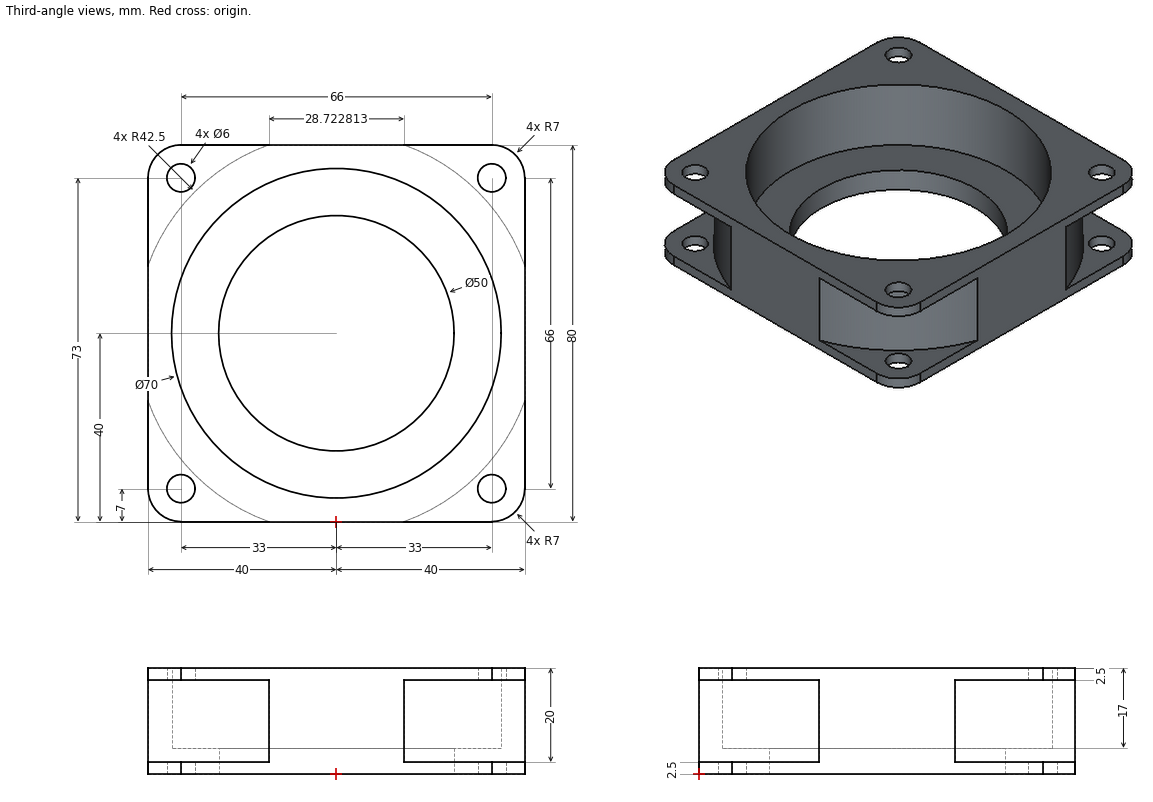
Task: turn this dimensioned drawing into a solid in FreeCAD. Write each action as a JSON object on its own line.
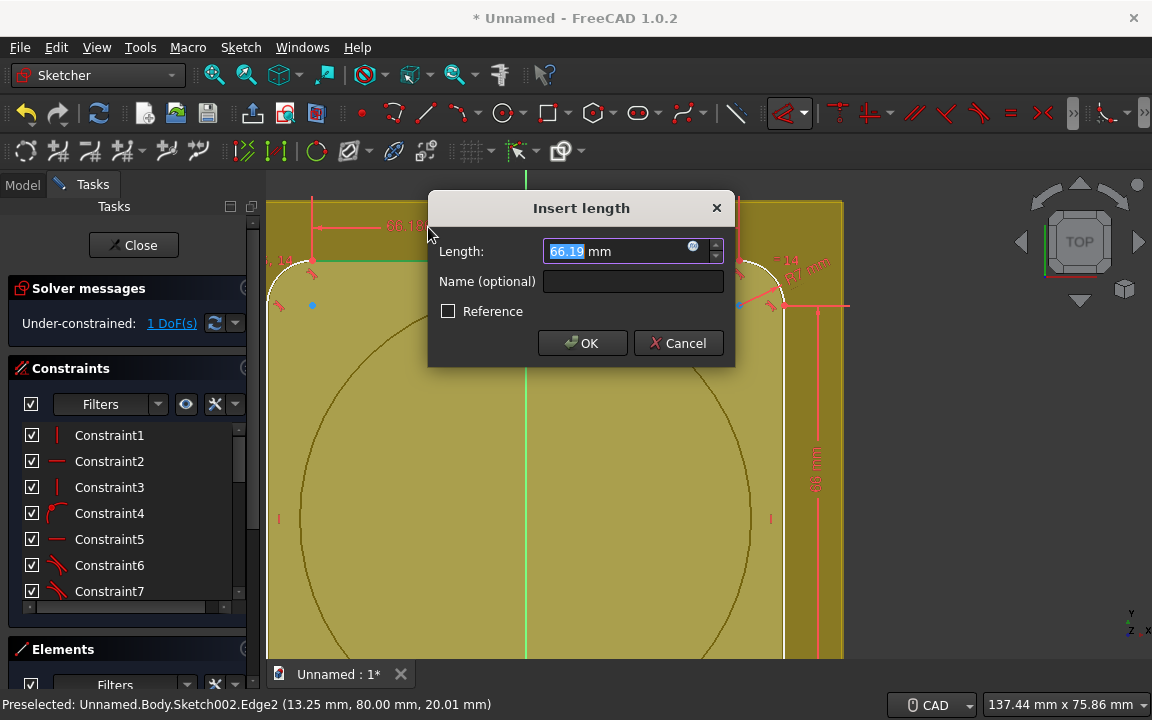
{"action": "type", "text": "66"}
{"action": "key", "text": "Return"}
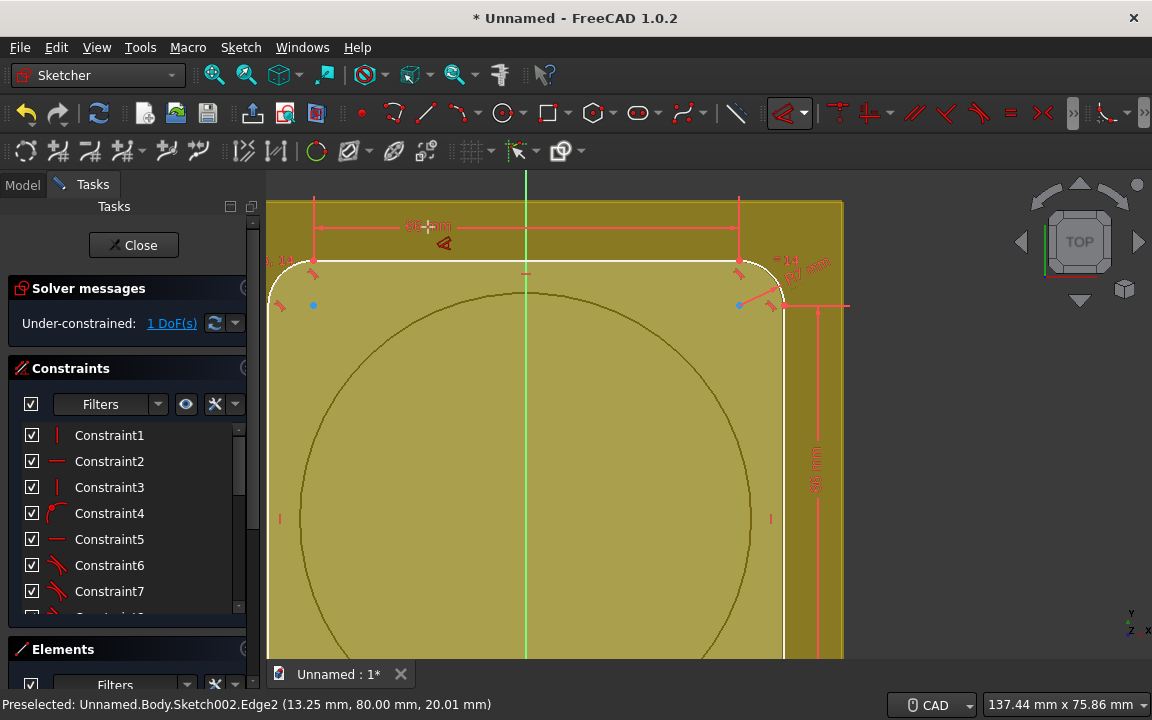
{"action": "scroll", "coordinate": [780, 288], "scroll_direction": "down", "scroll_amount": 3}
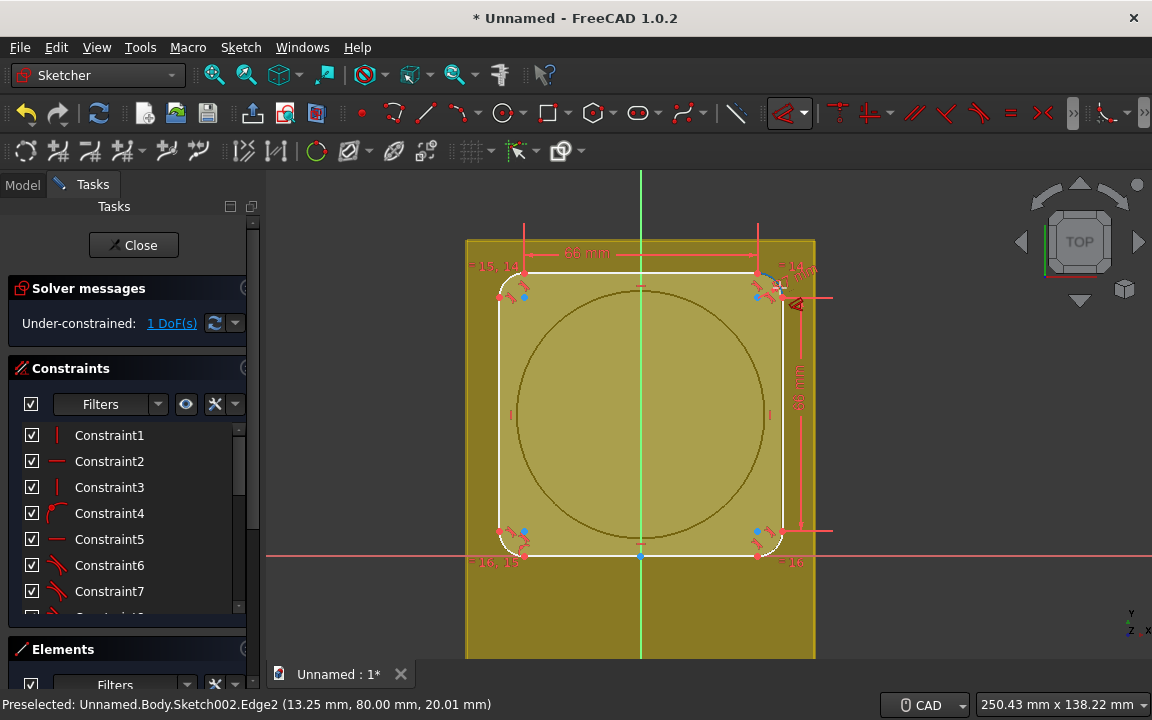
{"action": "left_click", "coordinate": [783, 531]}
{"action": "left_click", "coordinate": [712, 590]}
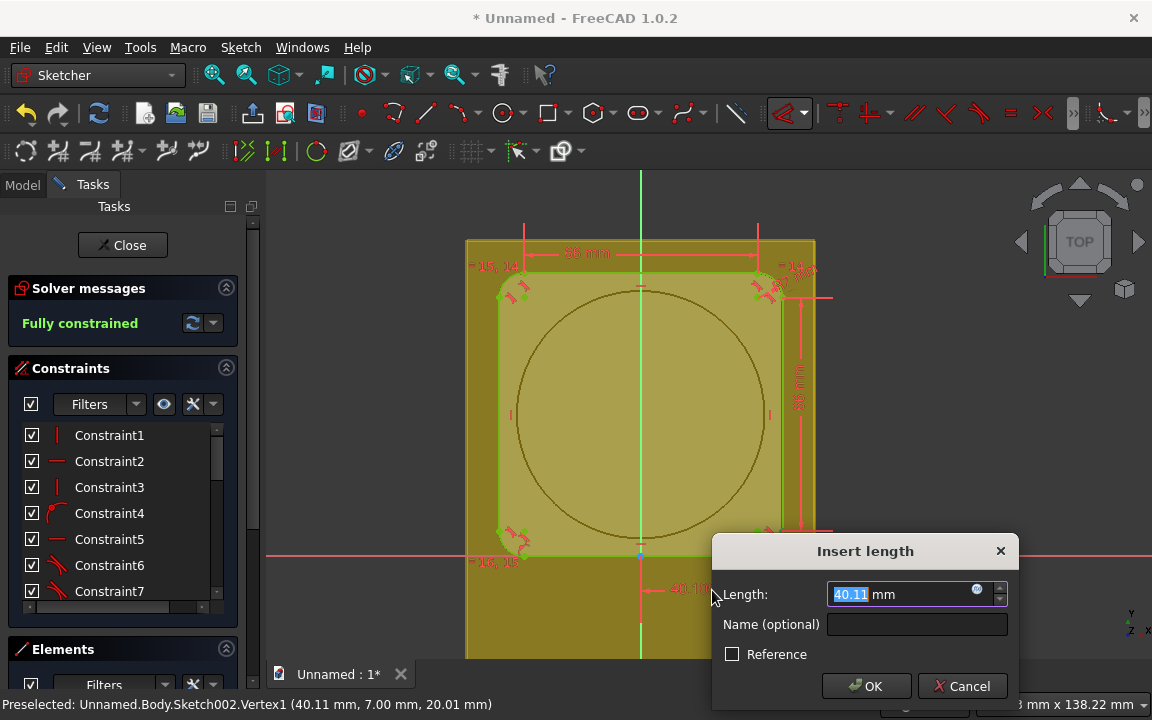
{"action": "type", "text": "40"}
{"action": "key", "text": "Return"}
{"action": "key", "text": "Escape"}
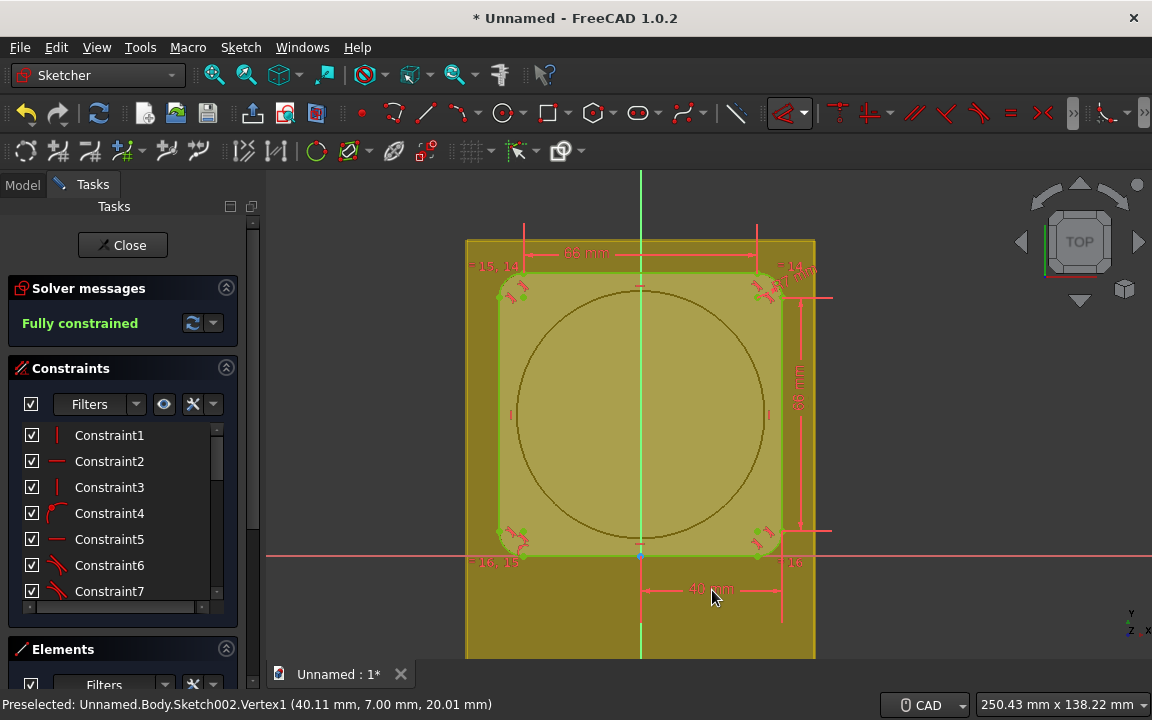
{"action": "left_click", "coordinate": [123, 245]}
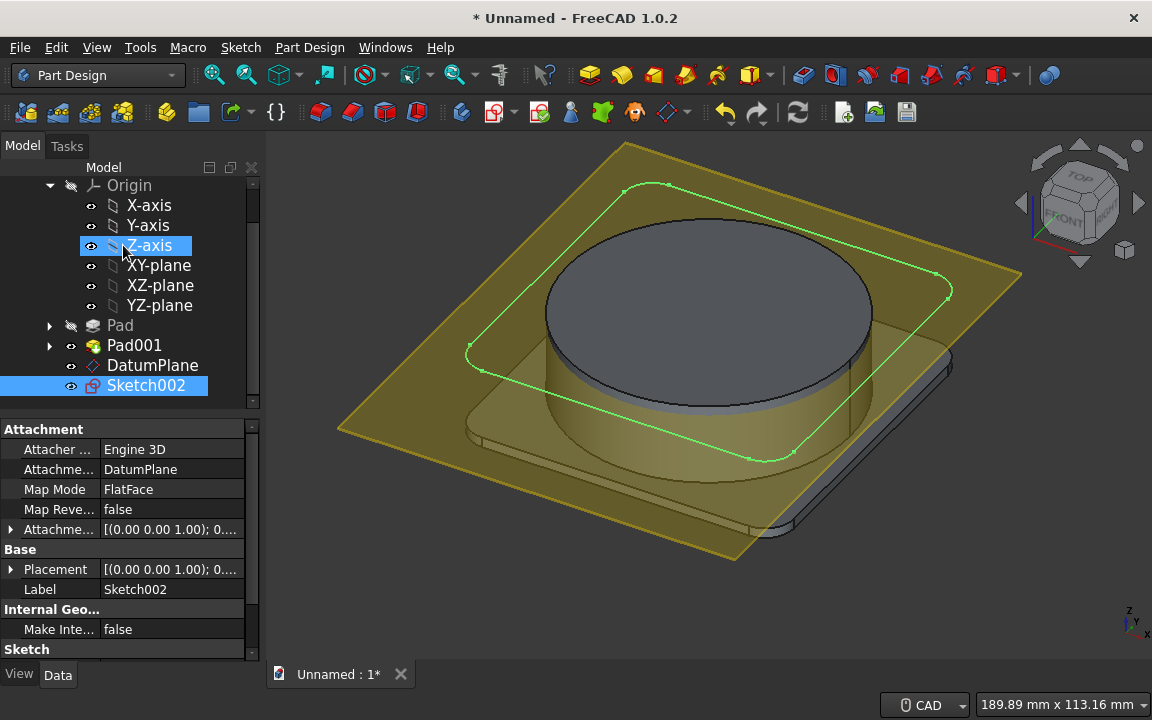
{"action": "left_click", "coordinate": [590, 76]}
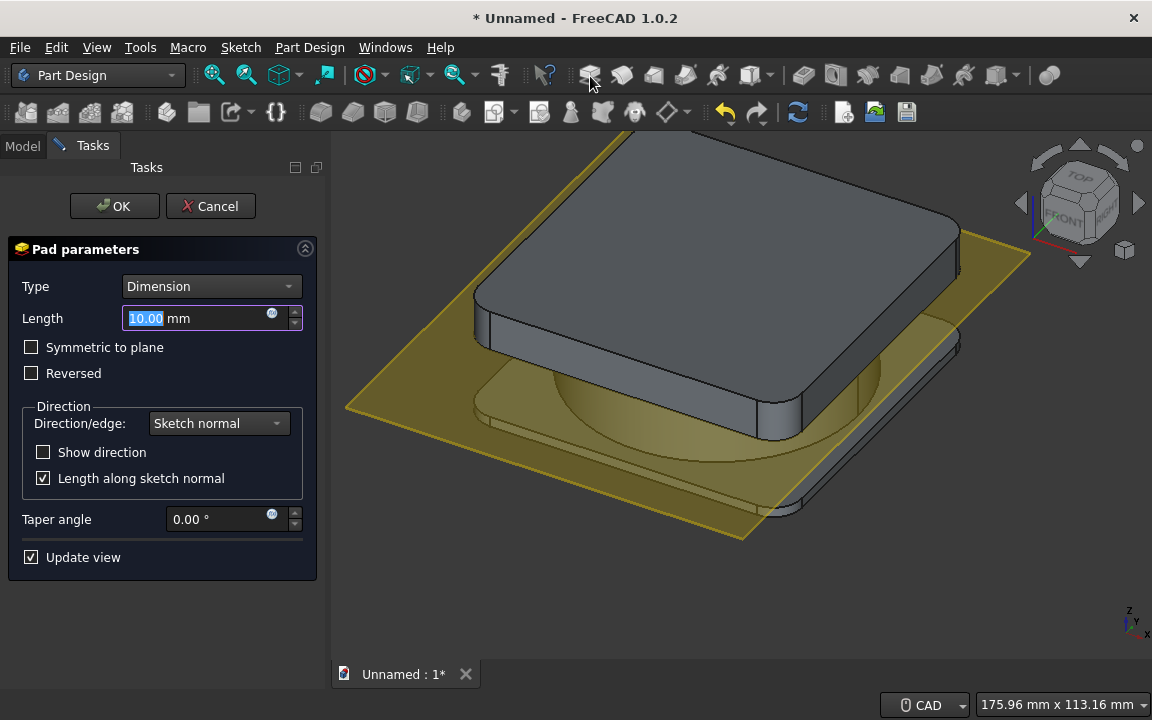
{"action": "type", "text": "2.5"}
{"action": "key", "text": "Tab"}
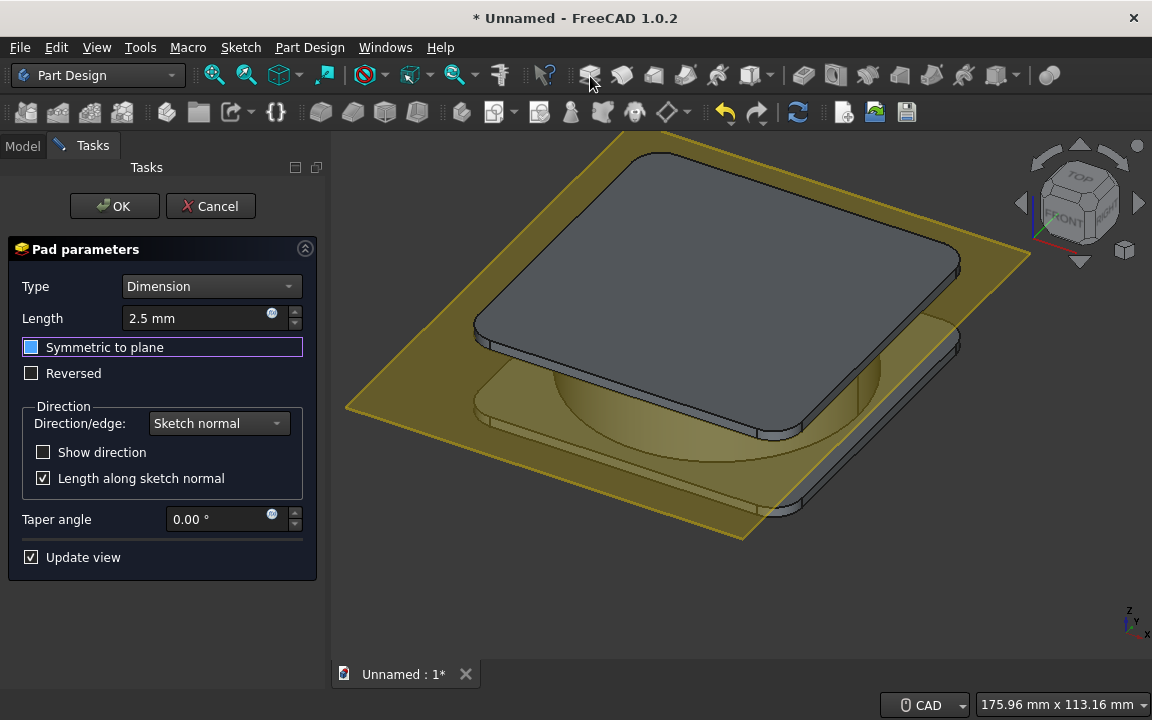
{"action": "left_click", "coordinate": [115, 206]}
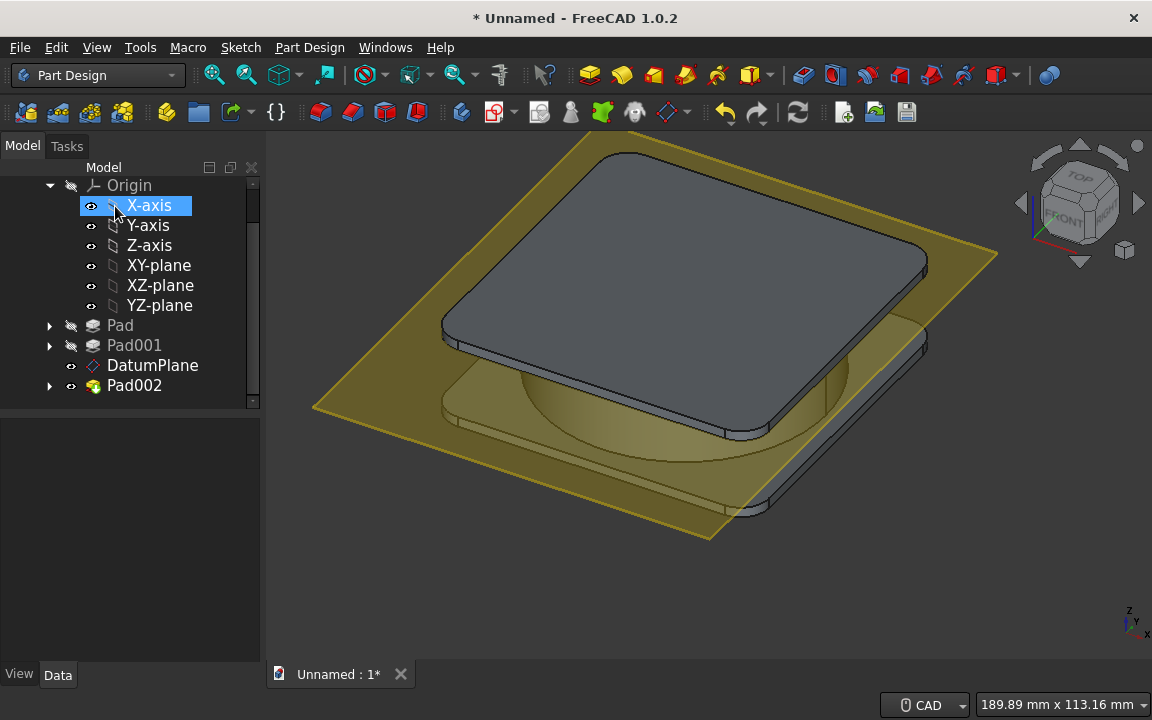
{"action": "left_click", "coordinate": [116, 366]}
{"action": "key", "text": "space"}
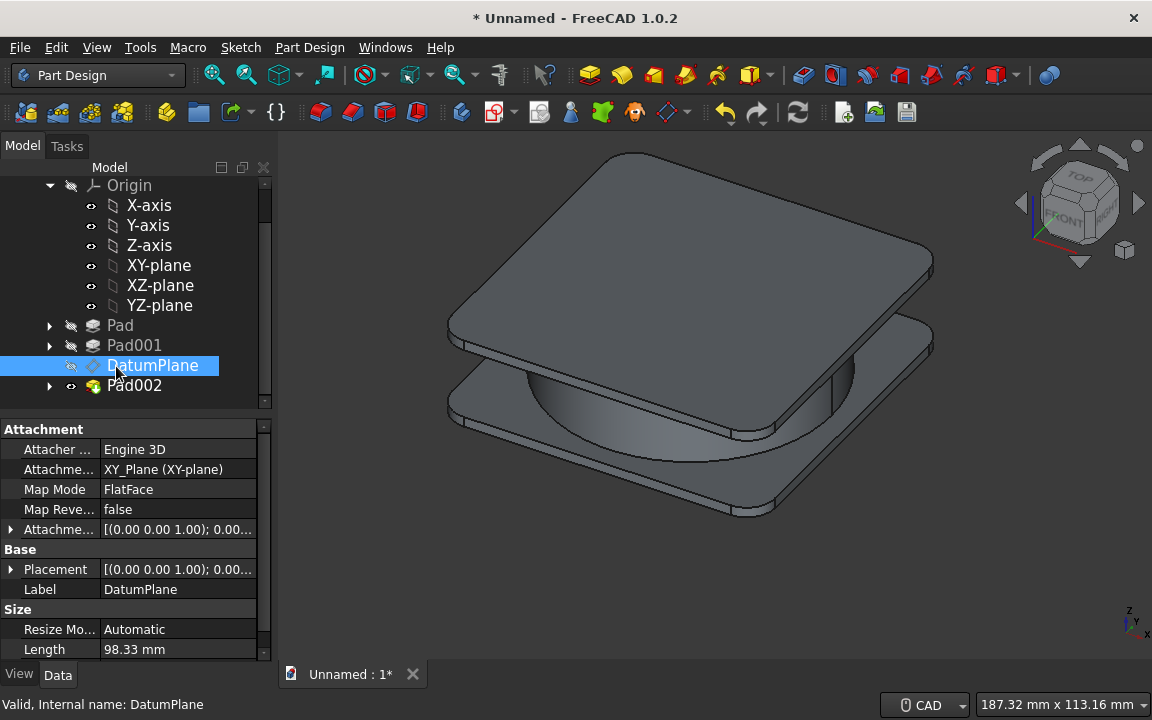
{"action": "left_click", "coordinate": [691, 291]}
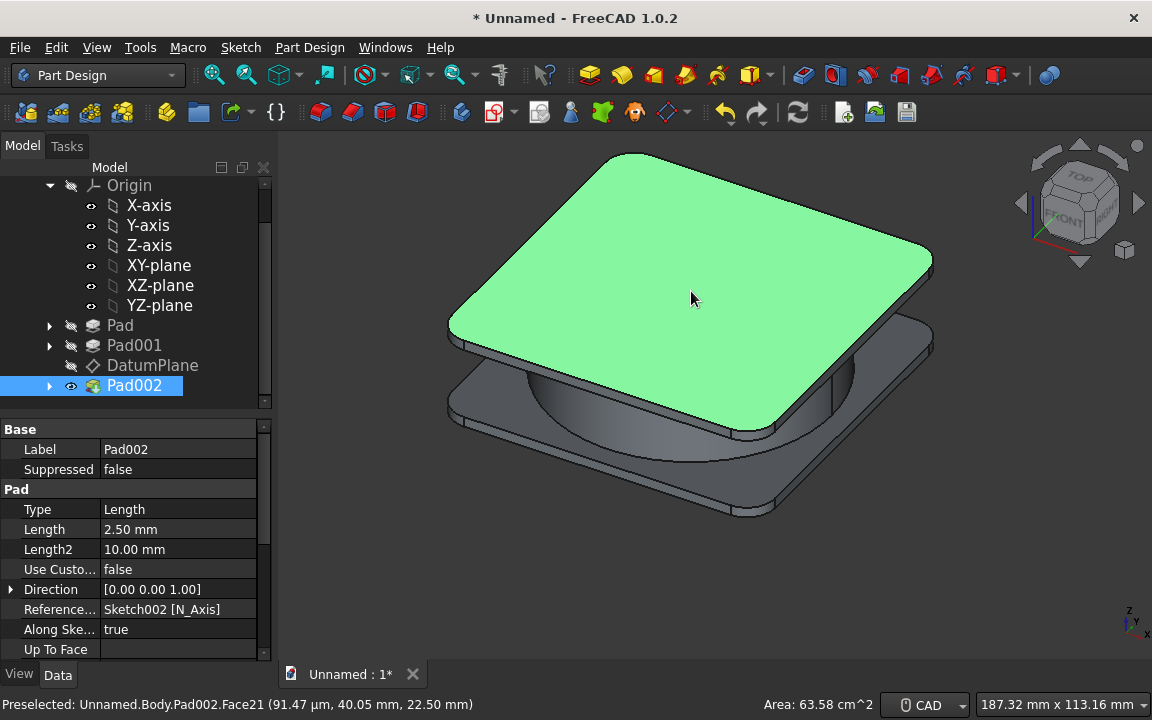
{"action": "left_click", "coordinate": [494, 112]}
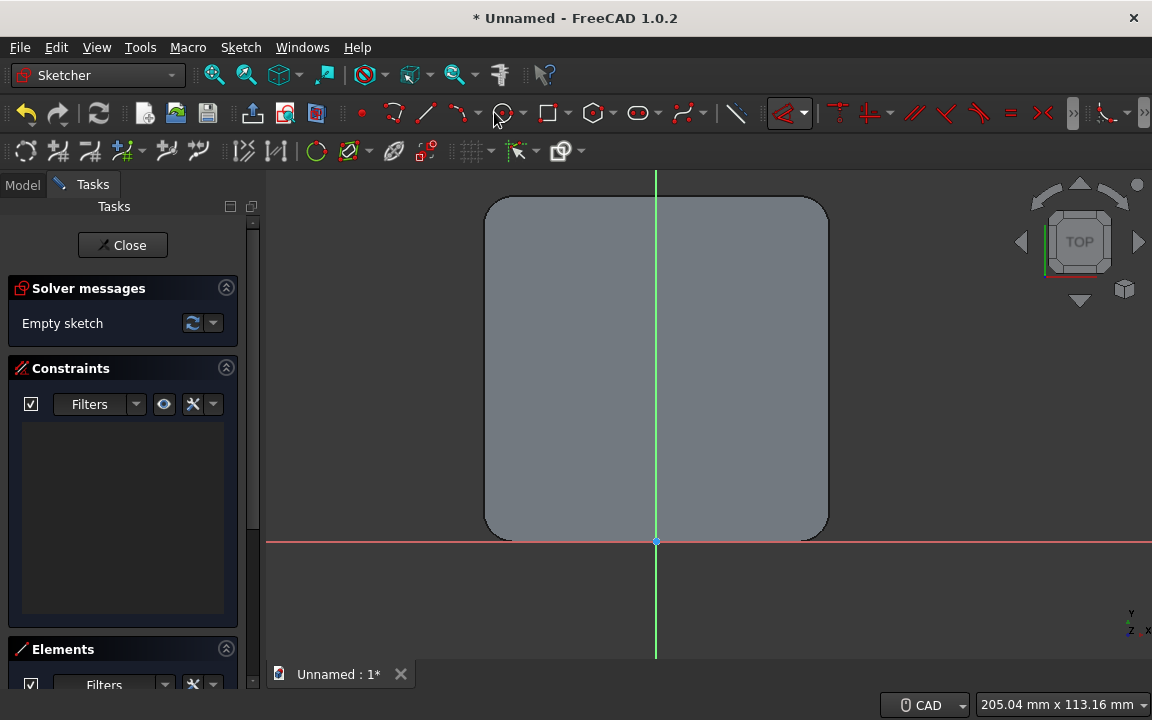
{"action": "scroll", "coordinate": [568, 621], "scroll_direction": "down", "scroll_amount": 1}